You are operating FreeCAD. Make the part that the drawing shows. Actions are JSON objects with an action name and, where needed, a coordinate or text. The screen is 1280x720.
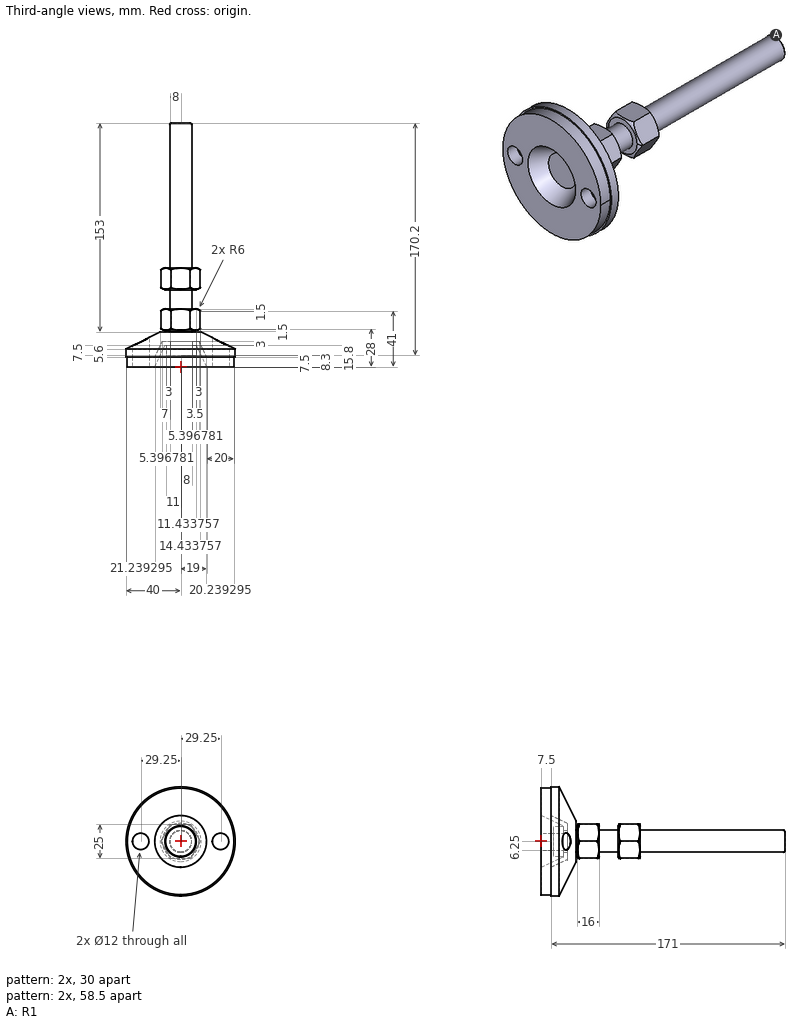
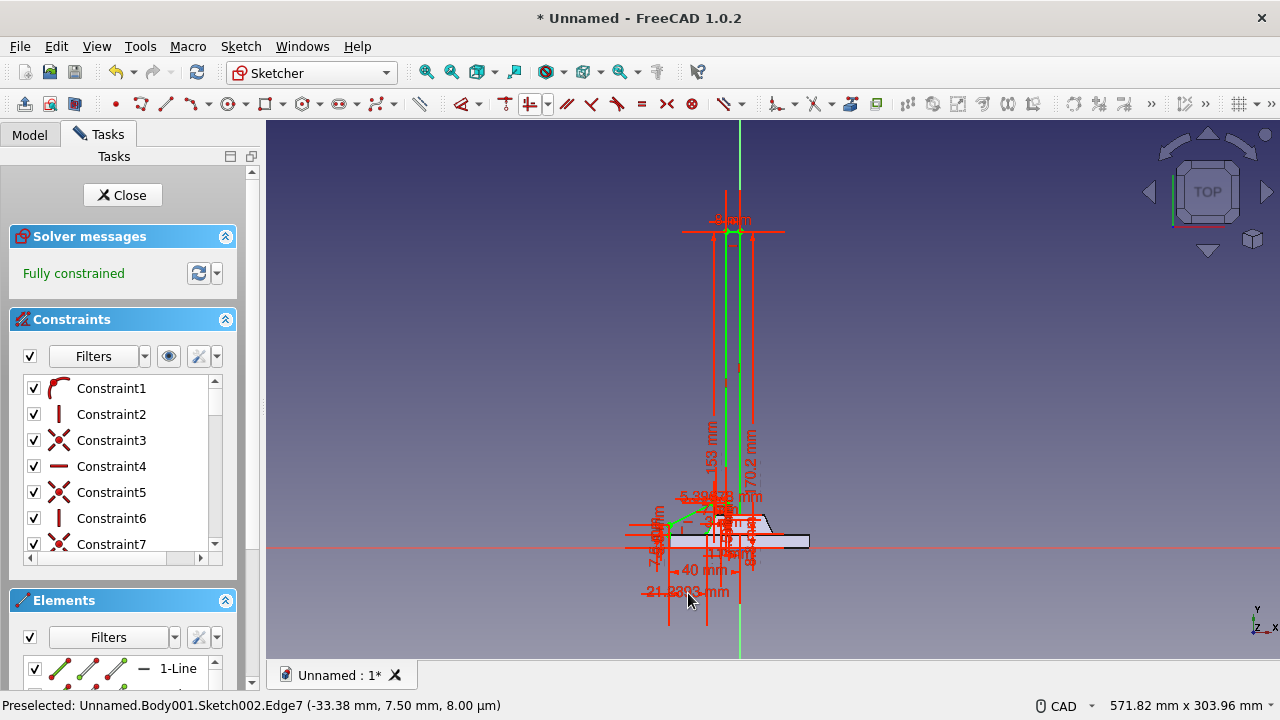
{"action": "left_click", "coordinate": [123, 195]}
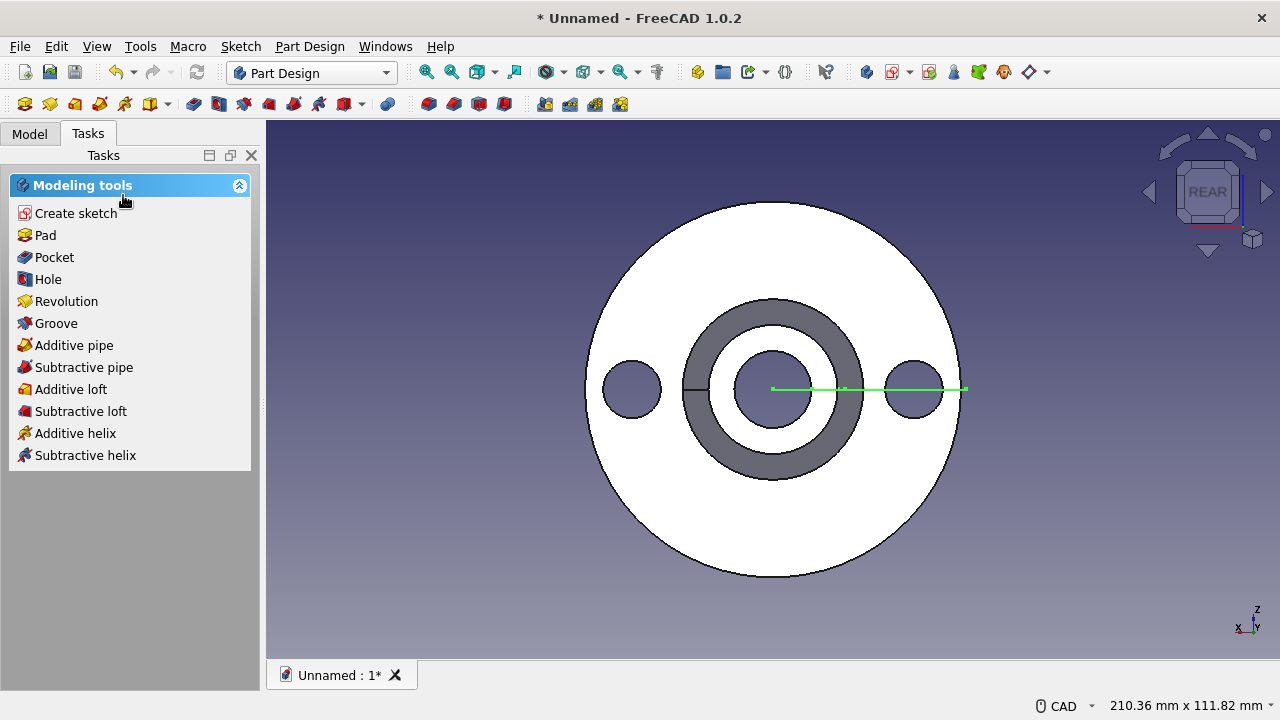
{"action": "left_click", "coordinate": [50, 104]}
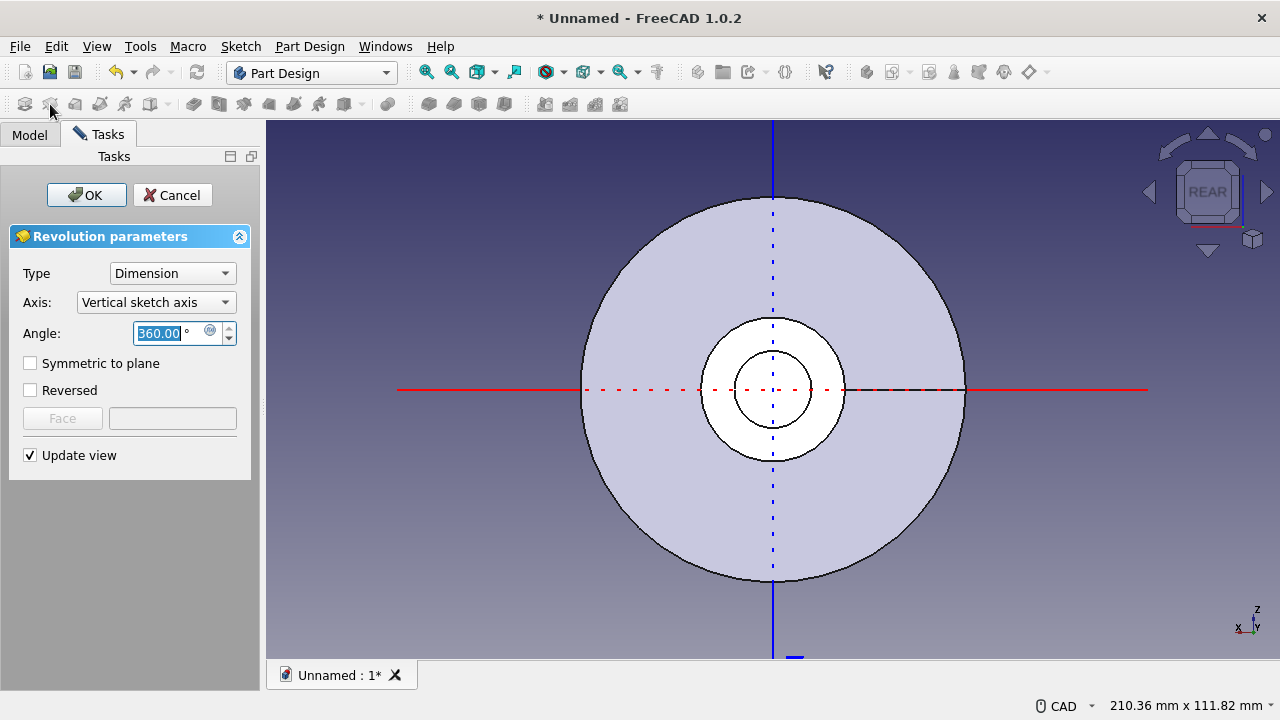
{"action": "left_click", "coordinate": [87, 195]}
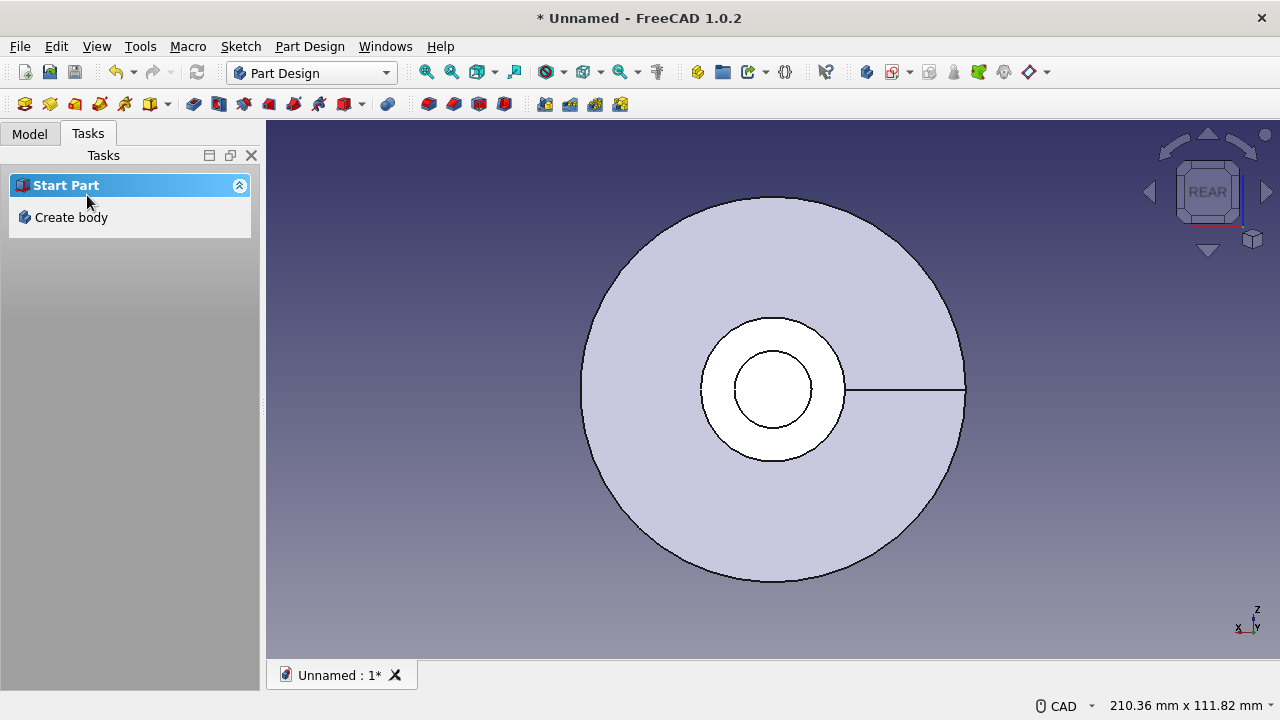
{"action": "left_click", "coordinate": [30, 134]}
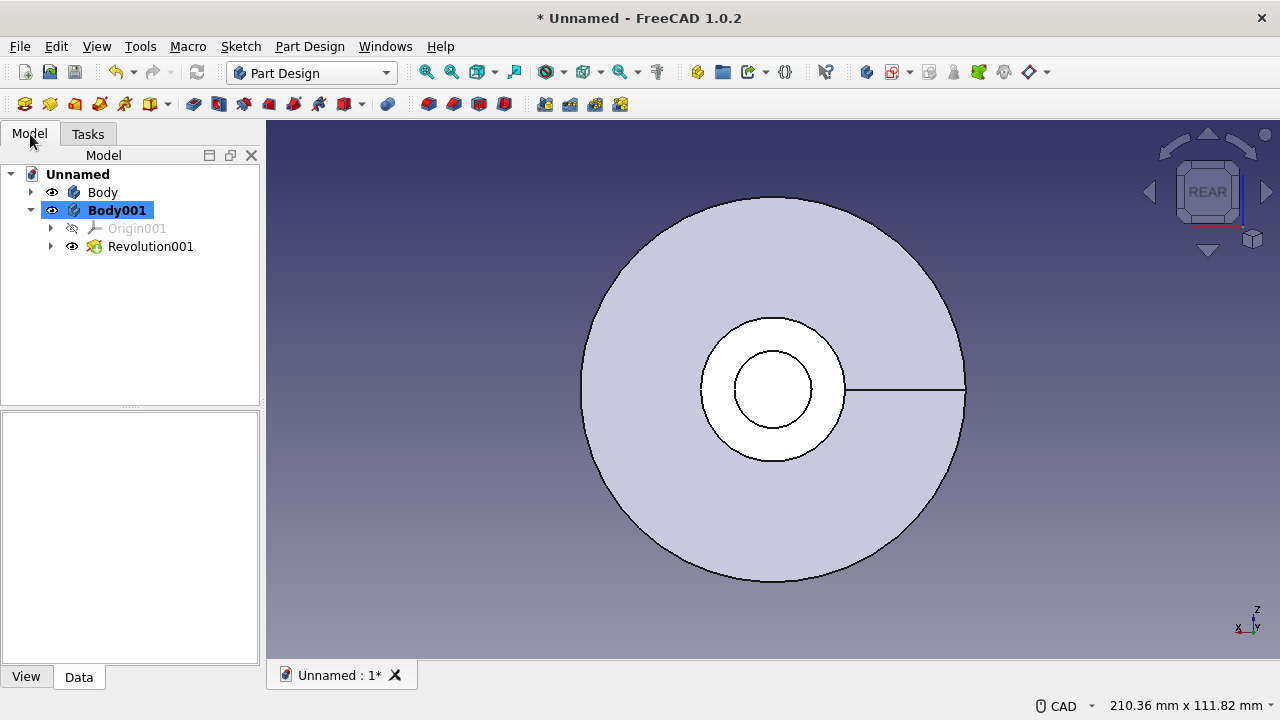
{"action": "left_click", "coordinate": [51, 228]}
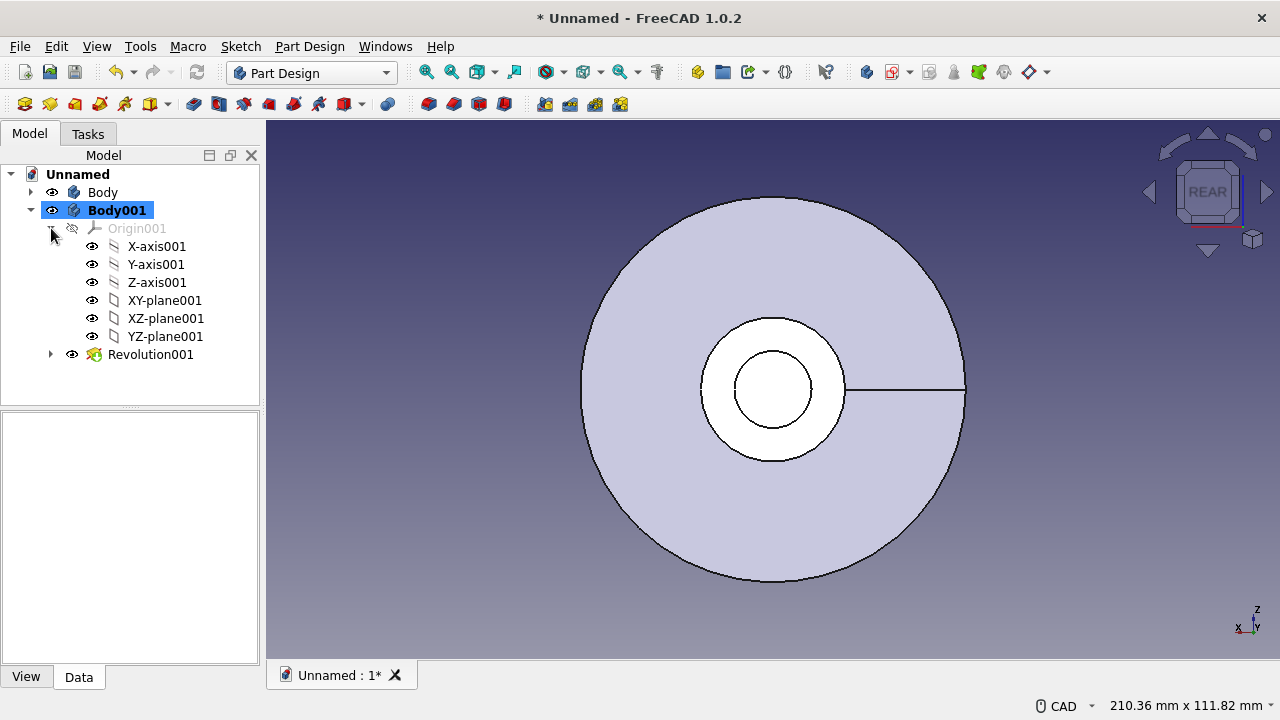
{"action": "left_click", "coordinate": [137, 318]}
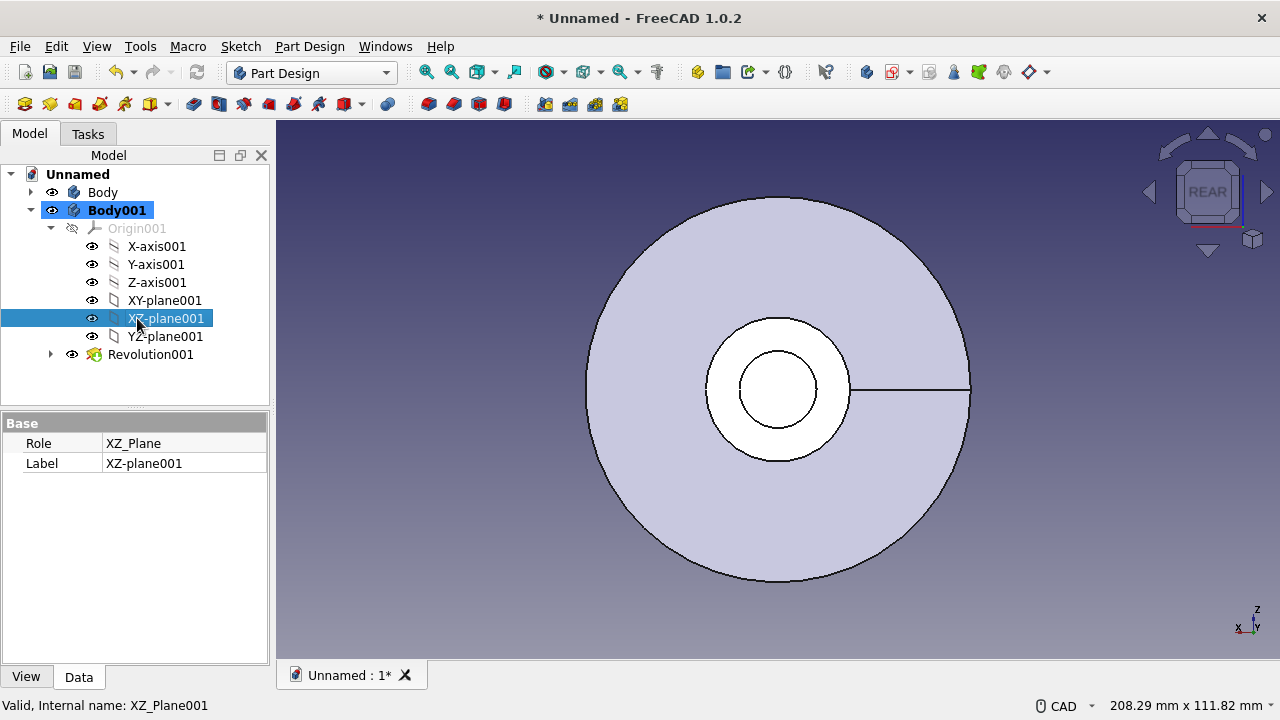
{"action": "left_click", "coordinate": [1028, 72]}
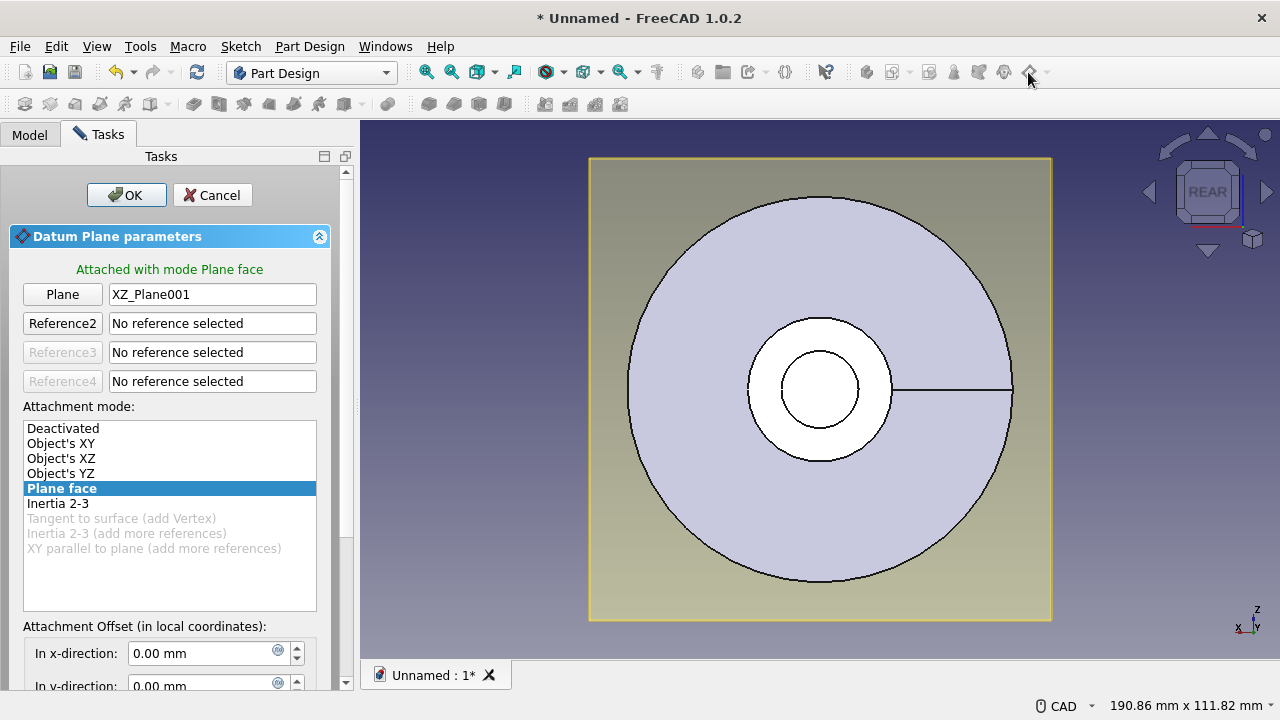
{"action": "scroll", "coordinate": [346, 428], "scroll_direction": "down", "scroll_amount": 2}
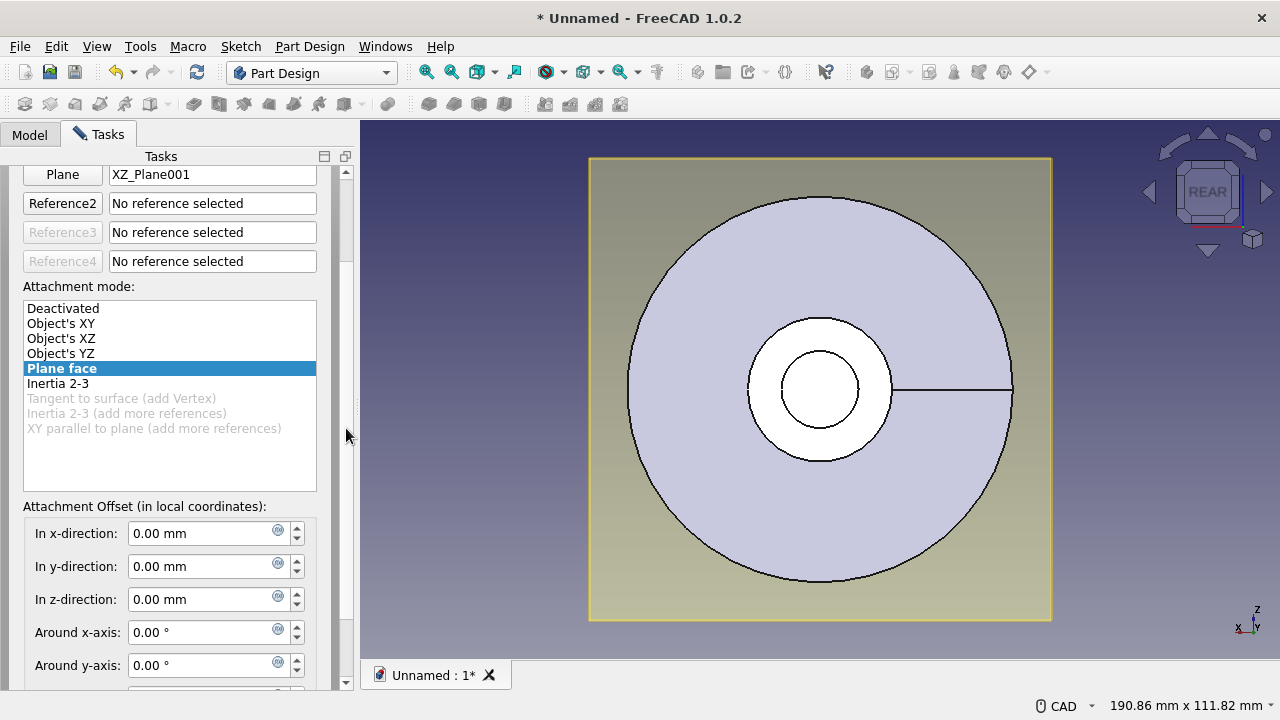
{"action": "triple_click", "coordinate": [210, 600]}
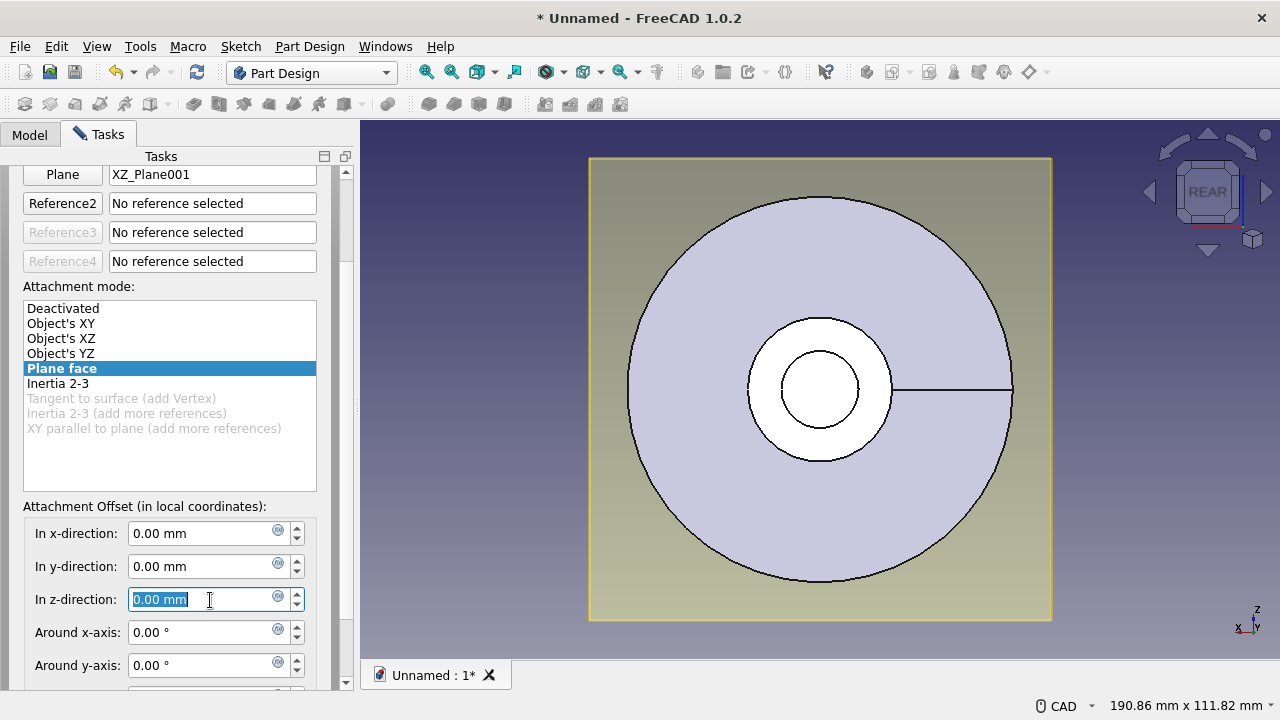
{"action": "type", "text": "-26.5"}
{"action": "key", "text": "Tab"}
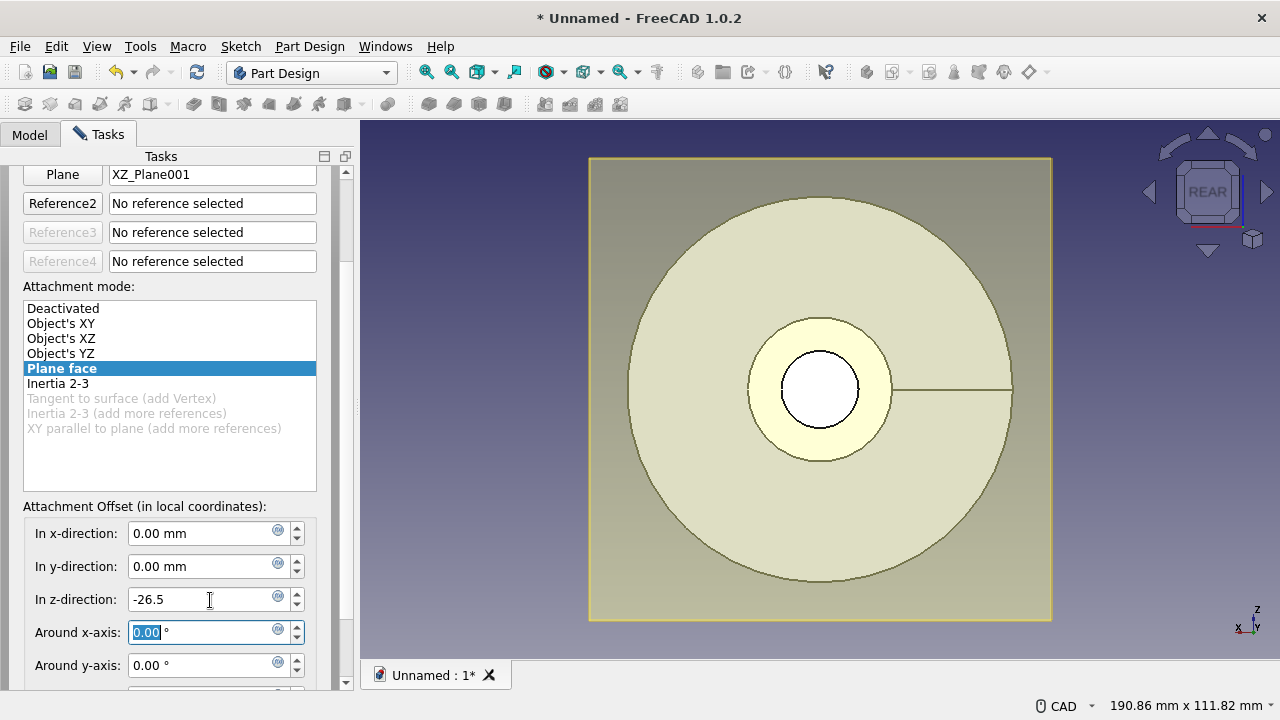
{"action": "scroll", "coordinate": [346, 428], "scroll_direction": "up", "scroll_amount": 3}